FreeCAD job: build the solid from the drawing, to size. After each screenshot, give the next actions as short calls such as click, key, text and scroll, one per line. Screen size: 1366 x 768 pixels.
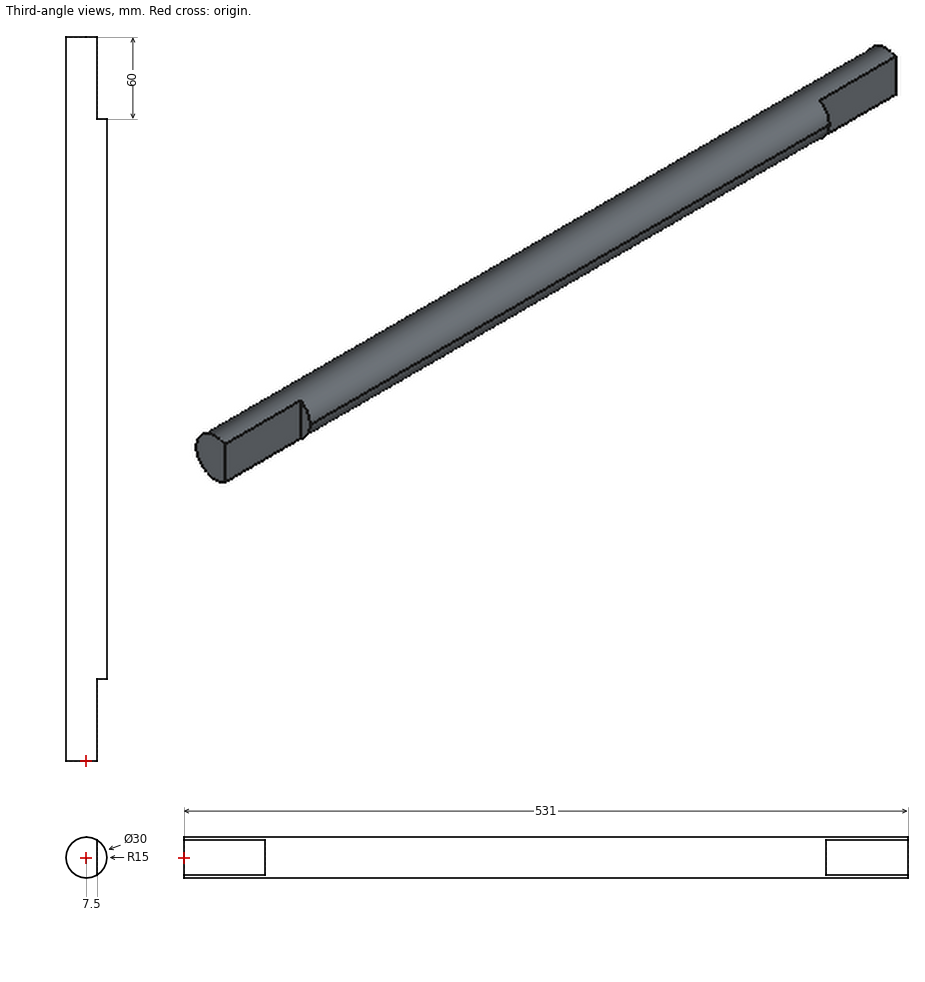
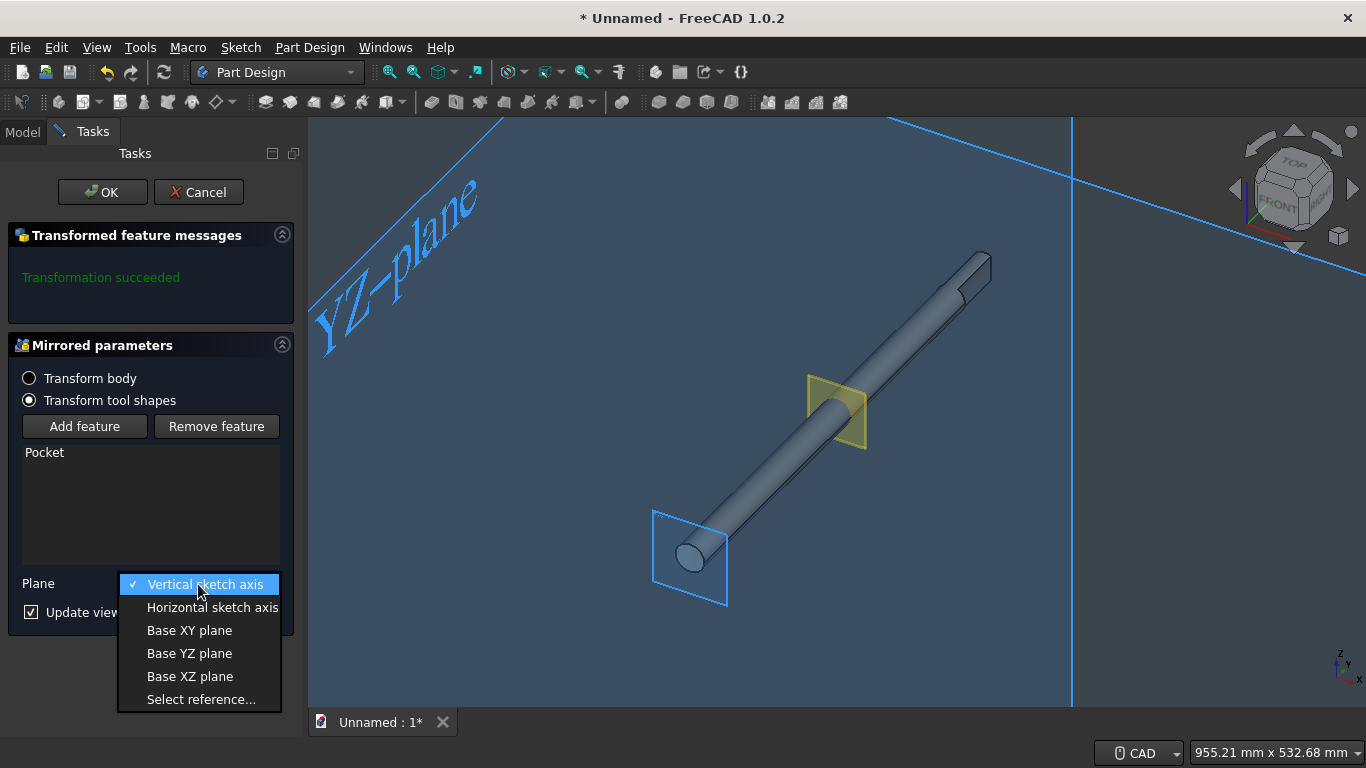
click(198, 700)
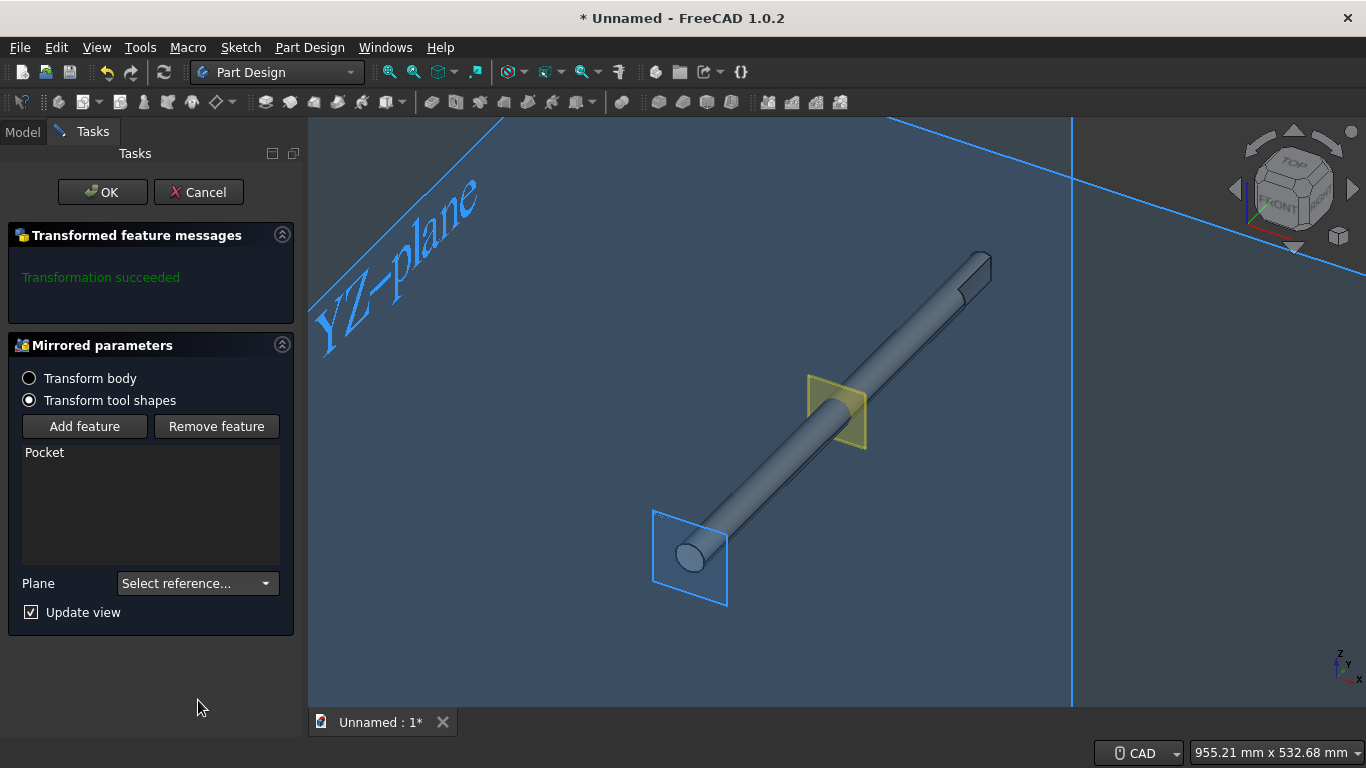
click(23, 131)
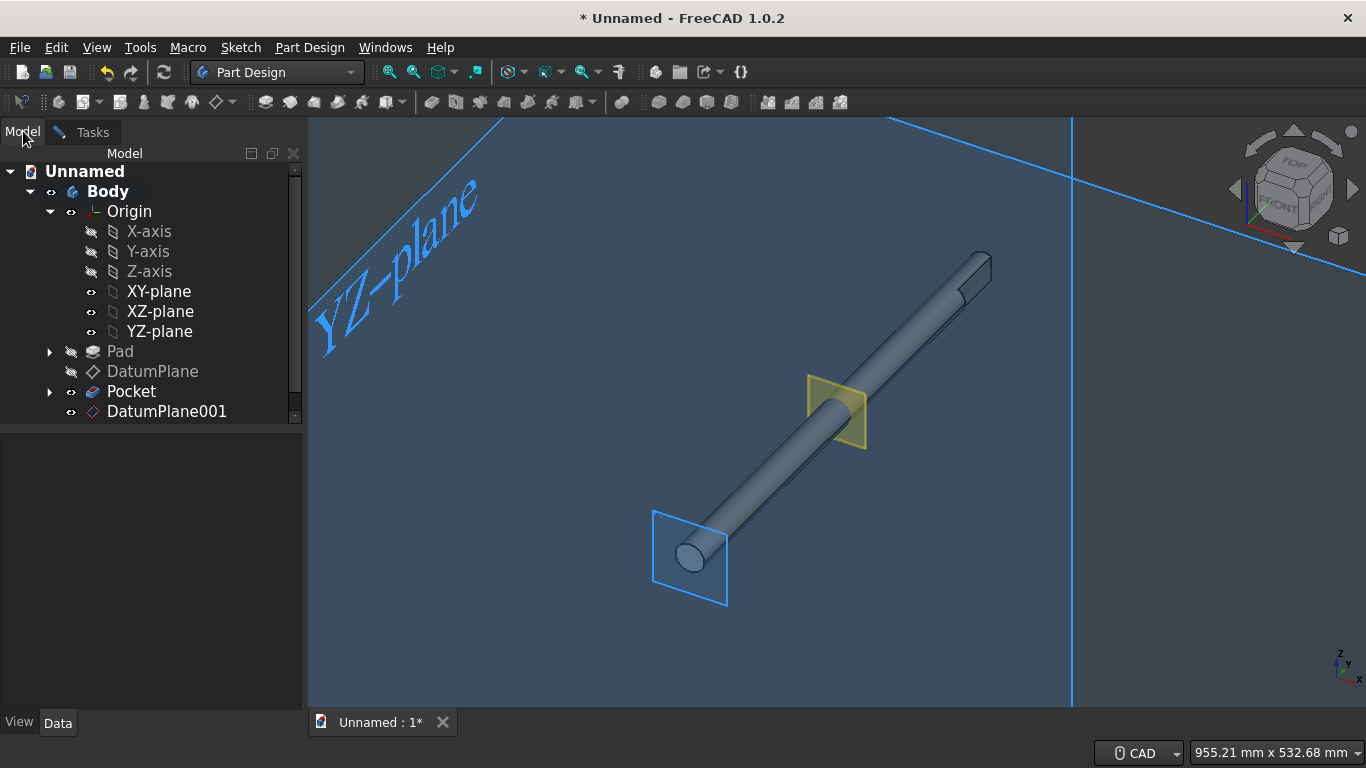
click(116, 412)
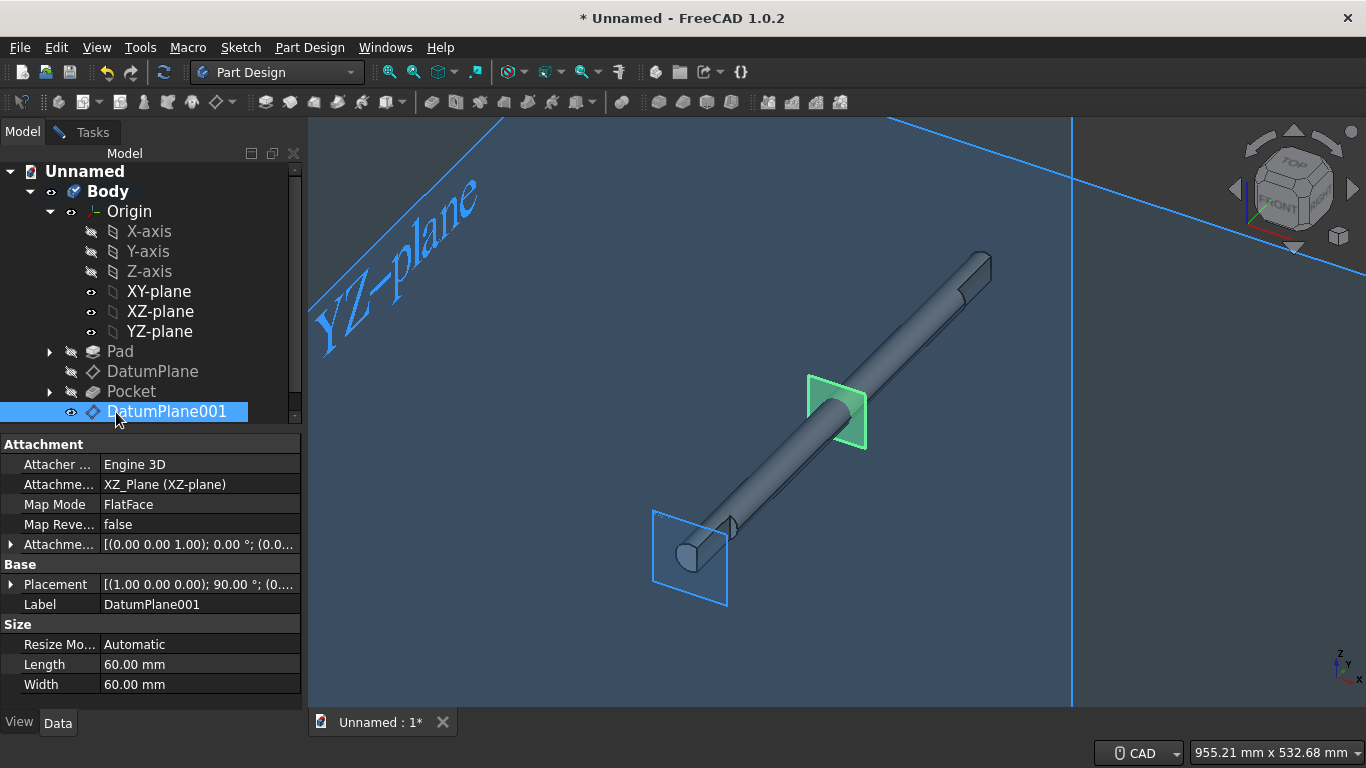
click(84, 131)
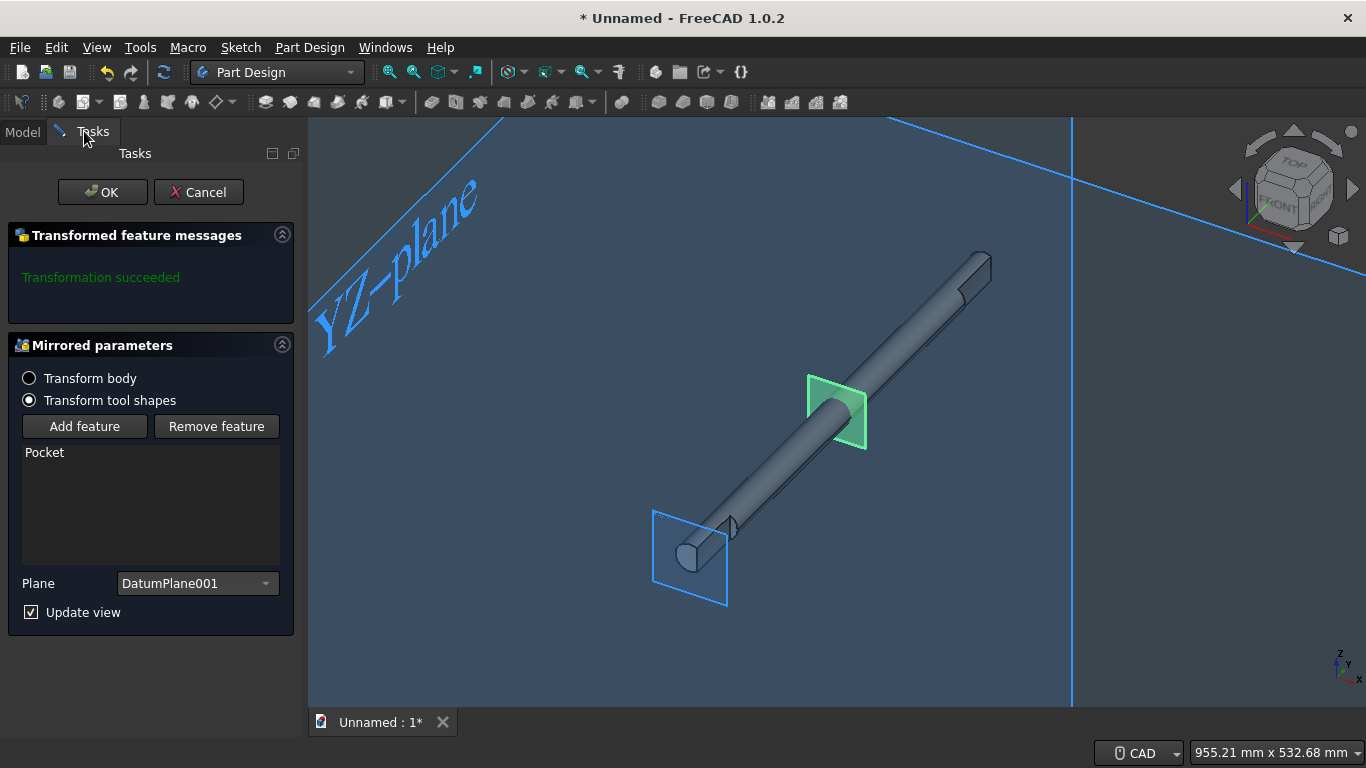
click(103, 192)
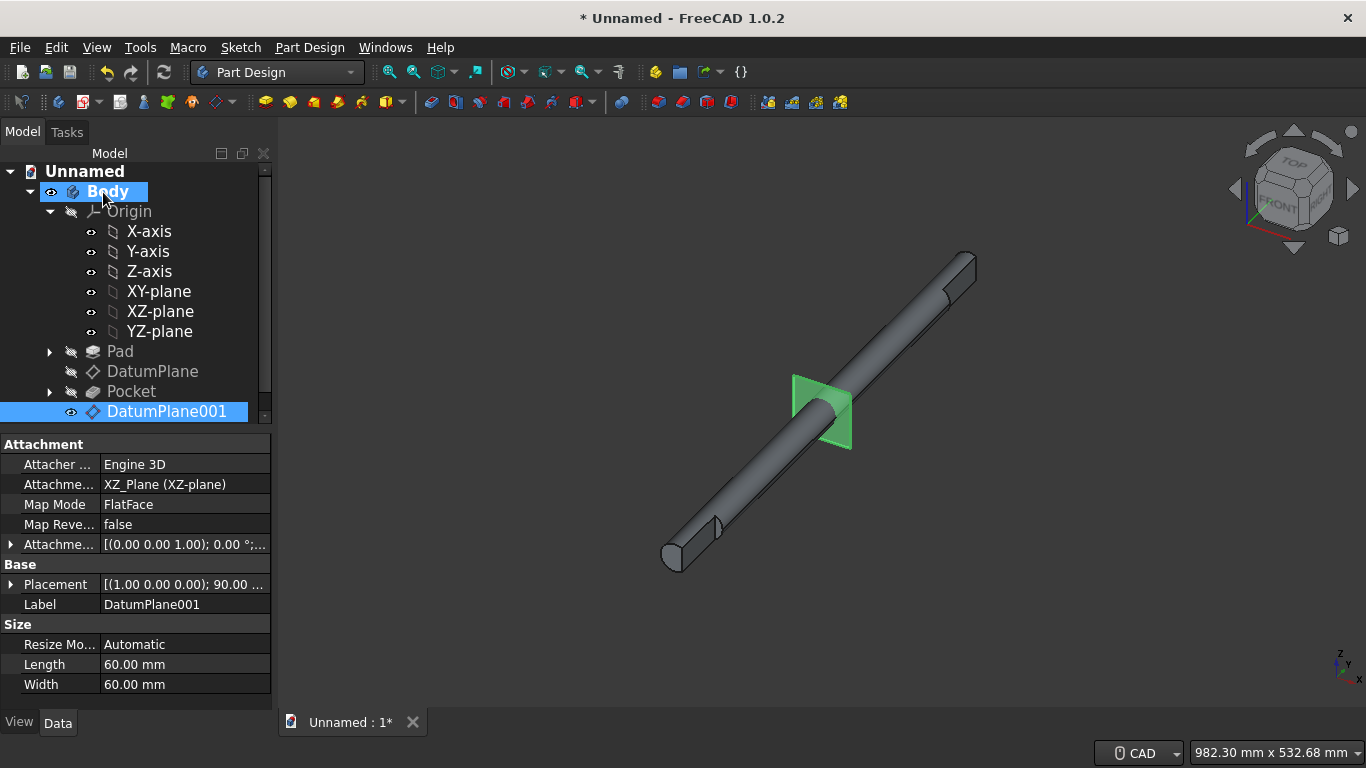
click(116, 412)
key(space)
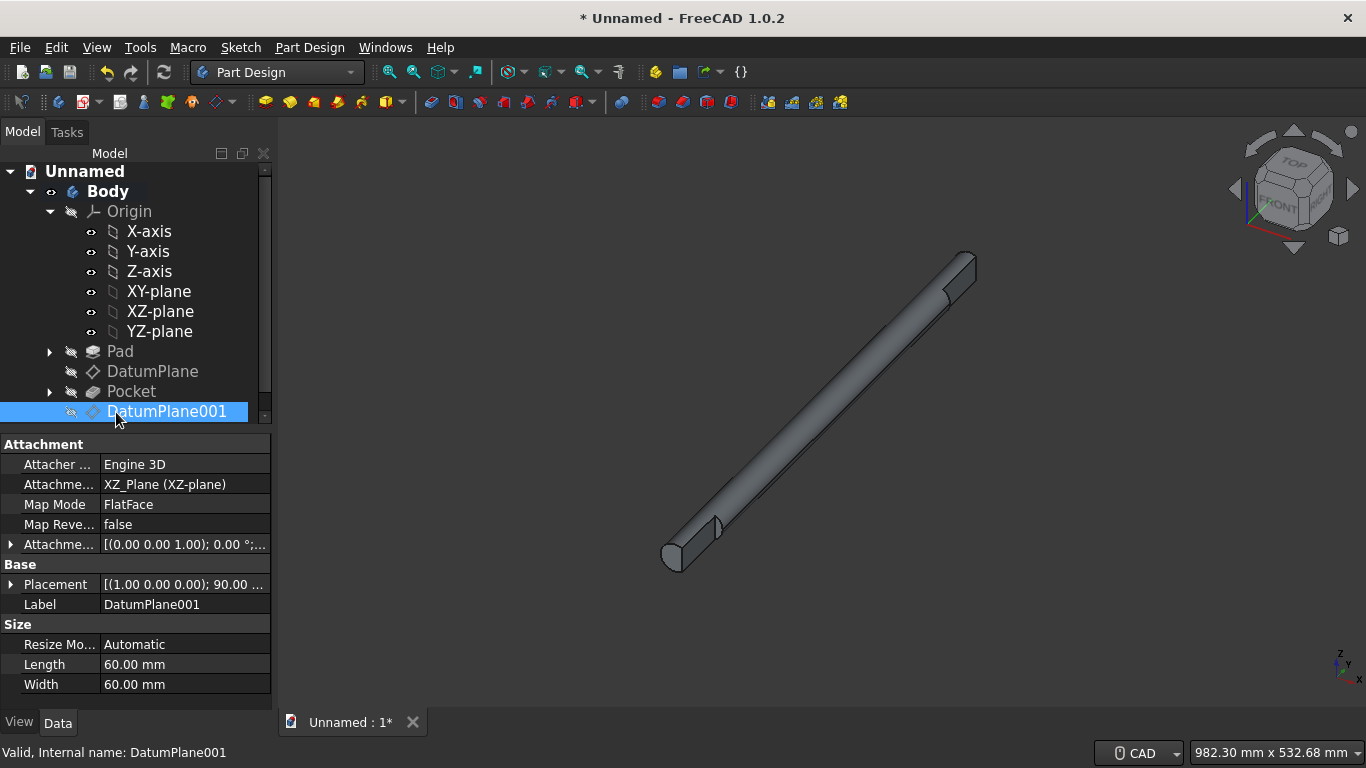
key(0)